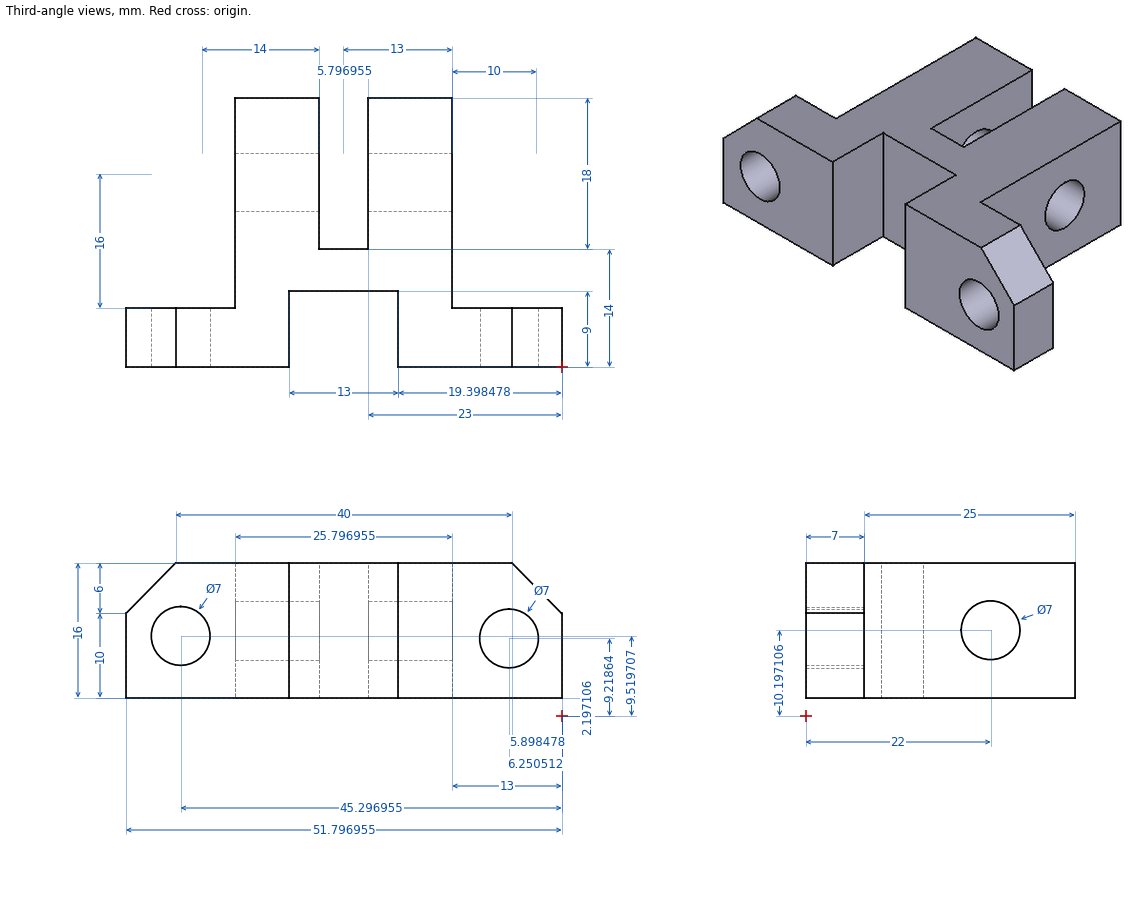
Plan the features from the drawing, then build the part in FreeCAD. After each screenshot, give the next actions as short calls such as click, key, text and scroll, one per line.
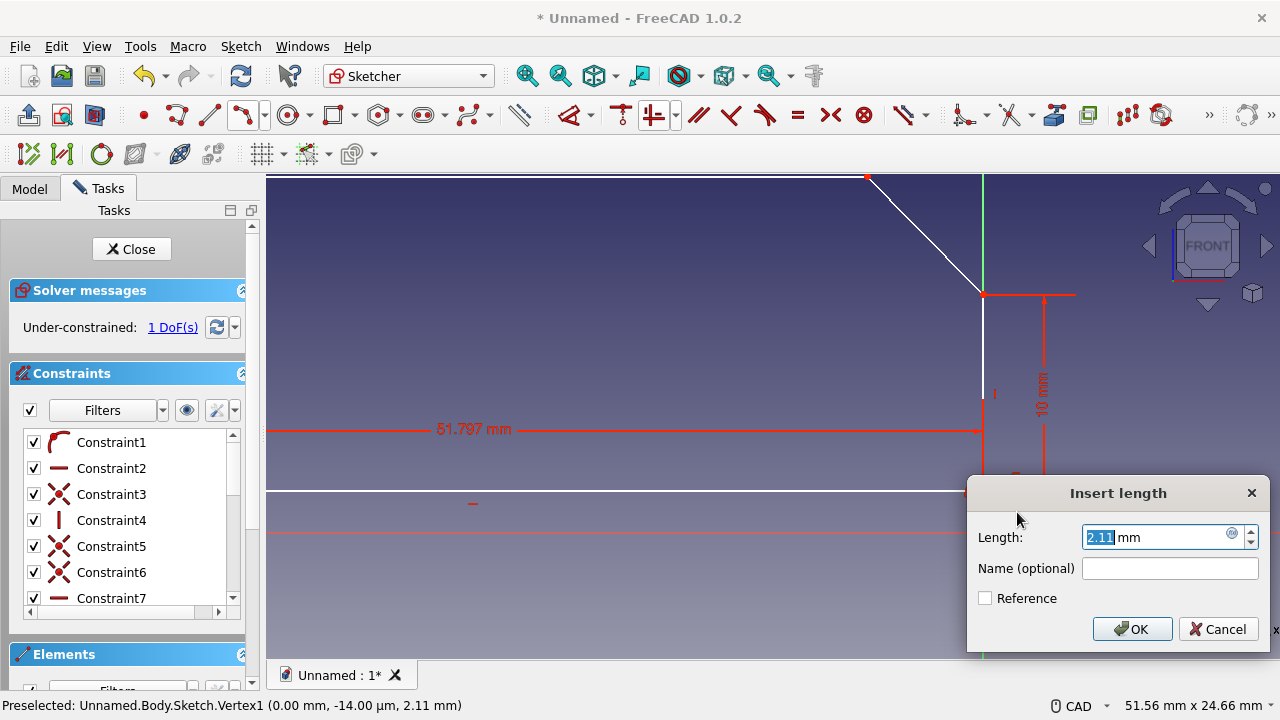
text(2.197106)
key(Return)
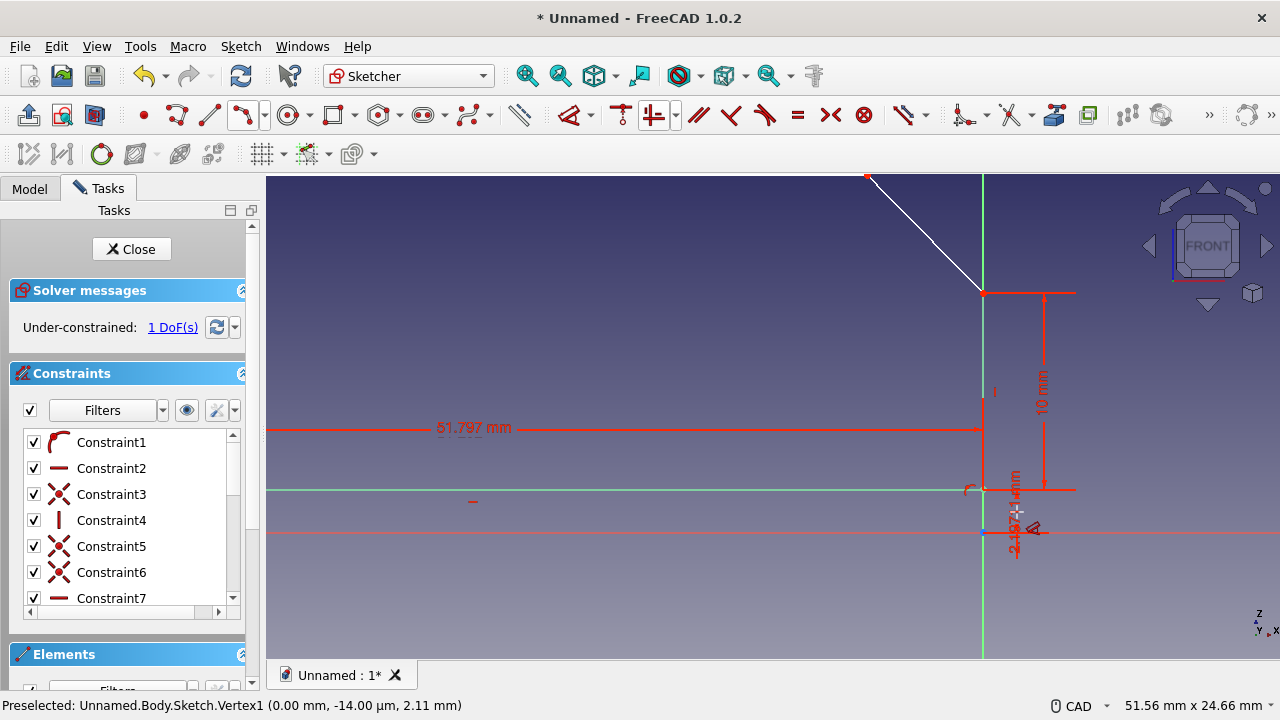
scroll(985, 493, down, 3)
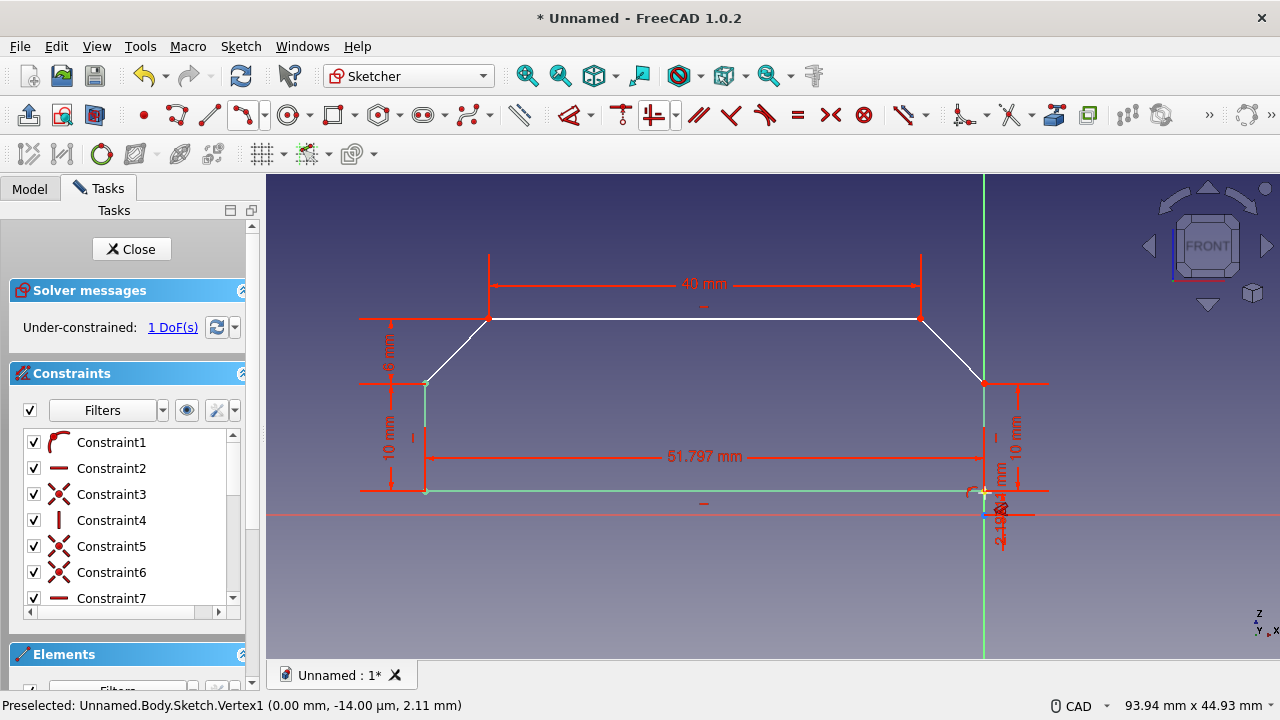
click(921, 319)
click(952, 549)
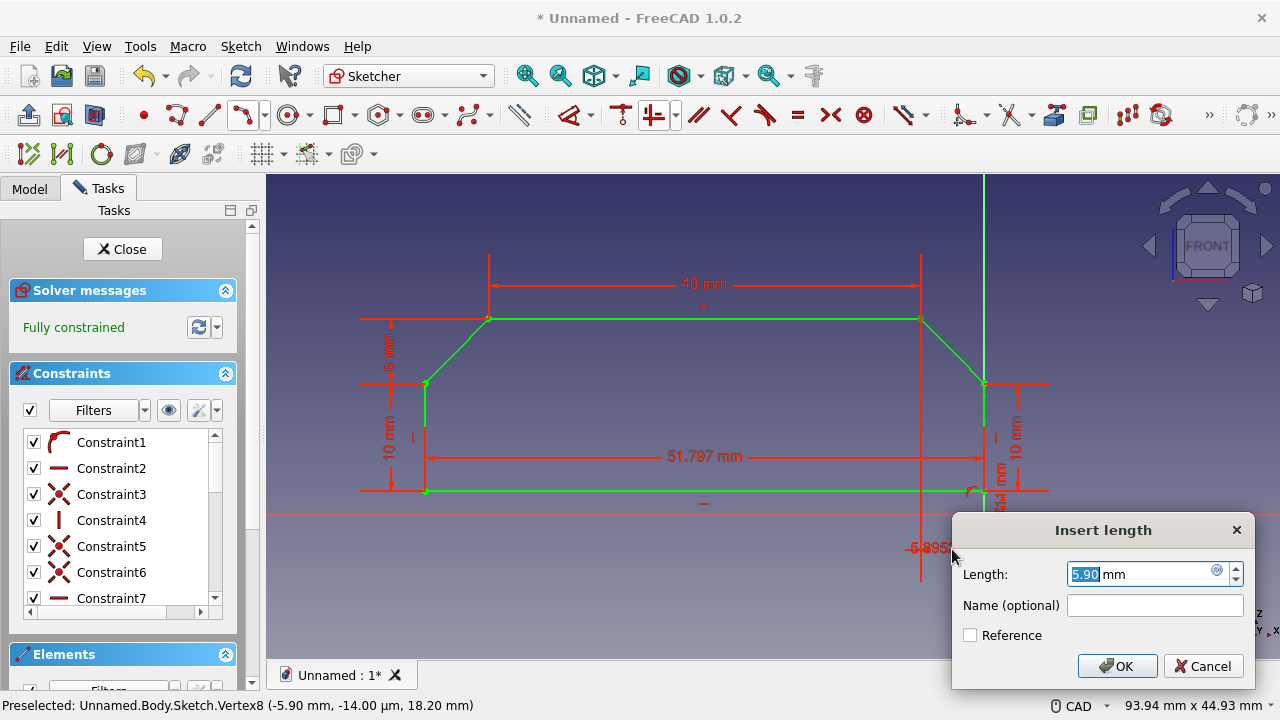
text(5.898478)
key(Return)
key(Escape)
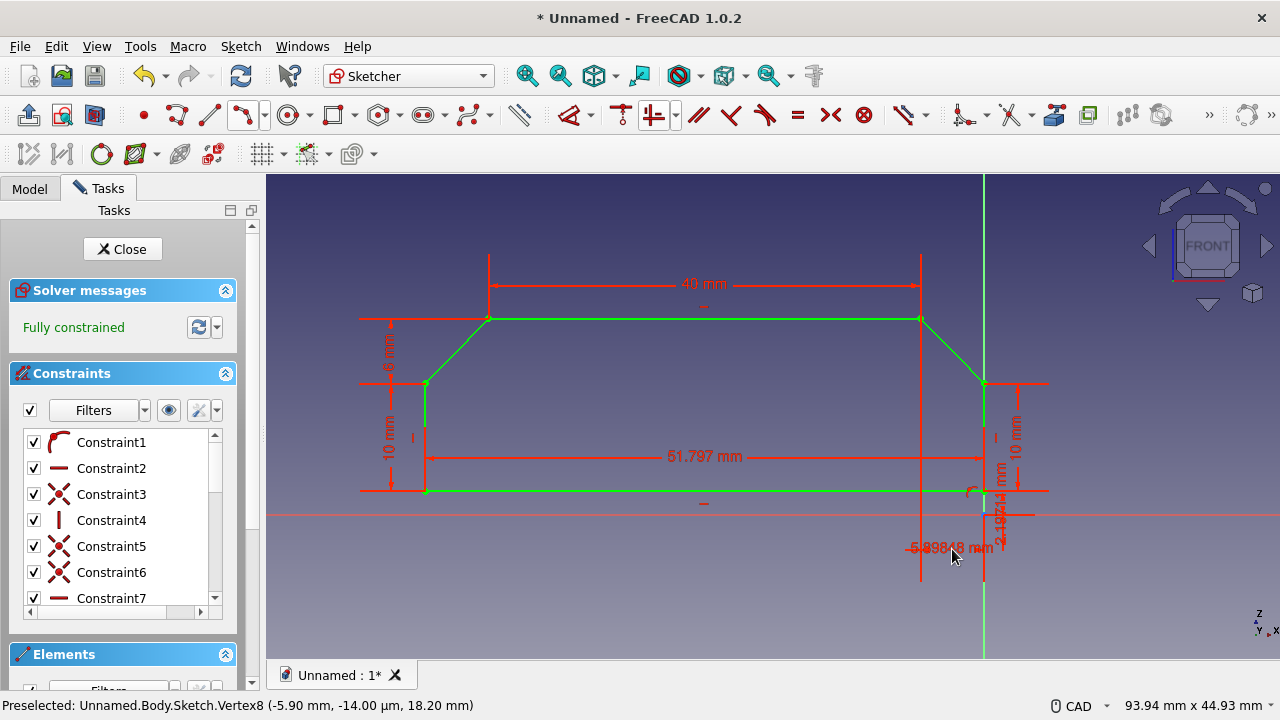
click(123, 249)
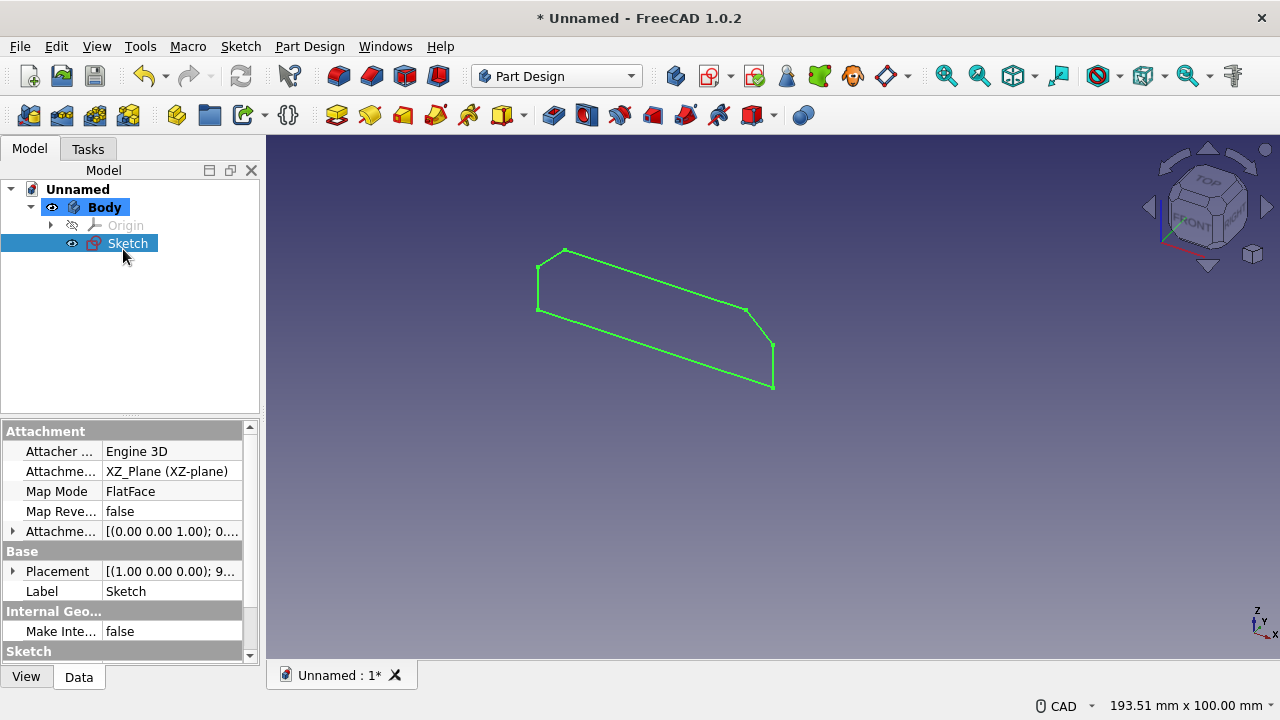
click(337, 116)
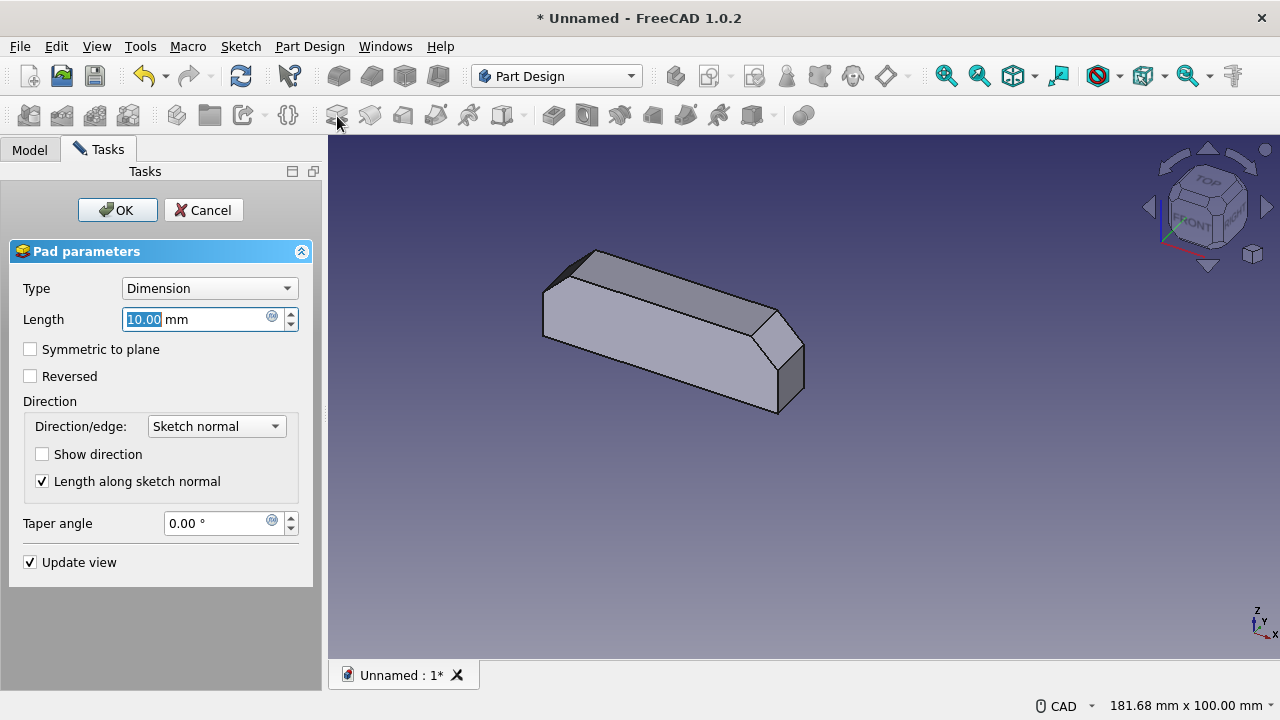
text(7)
key(Tab)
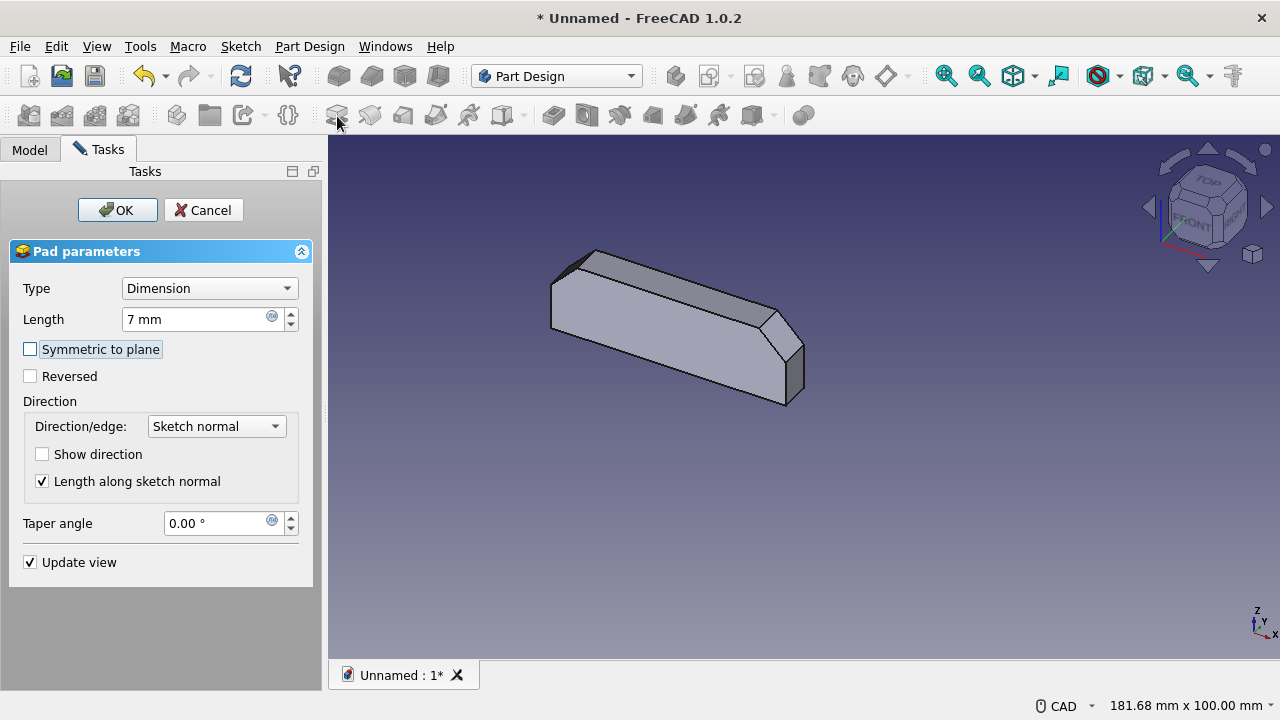
click(31, 376)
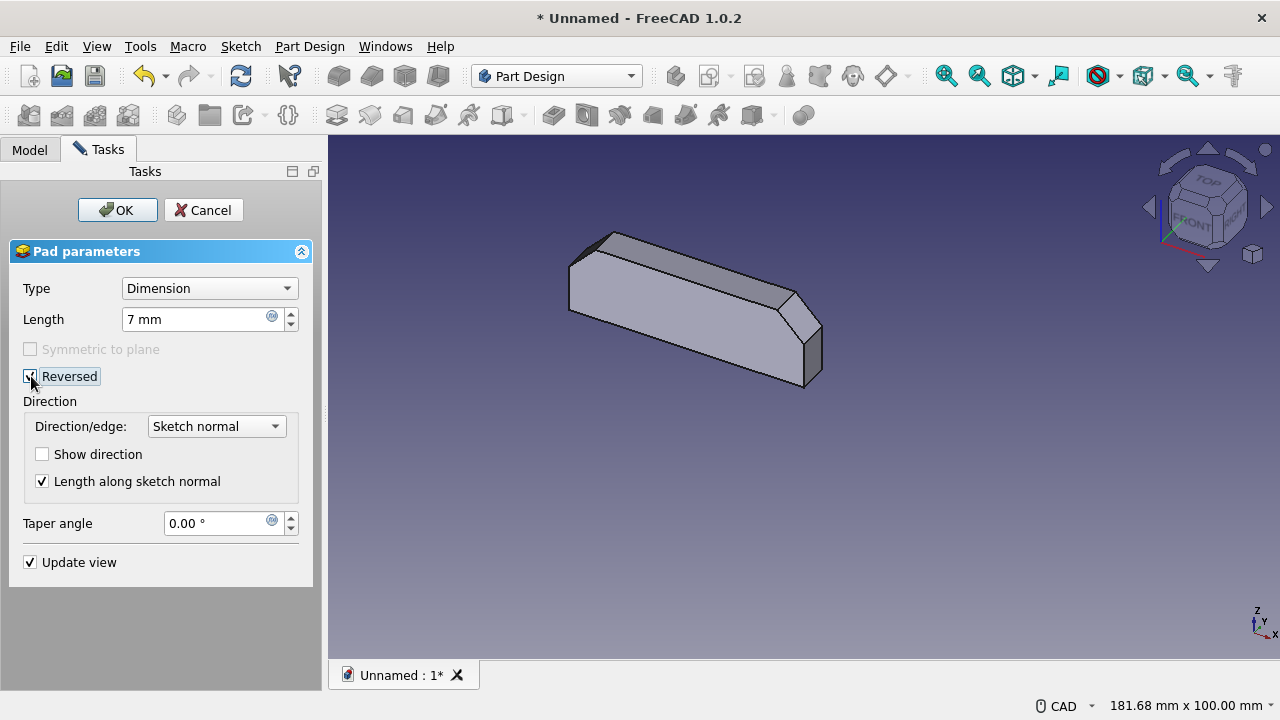
click(118, 210)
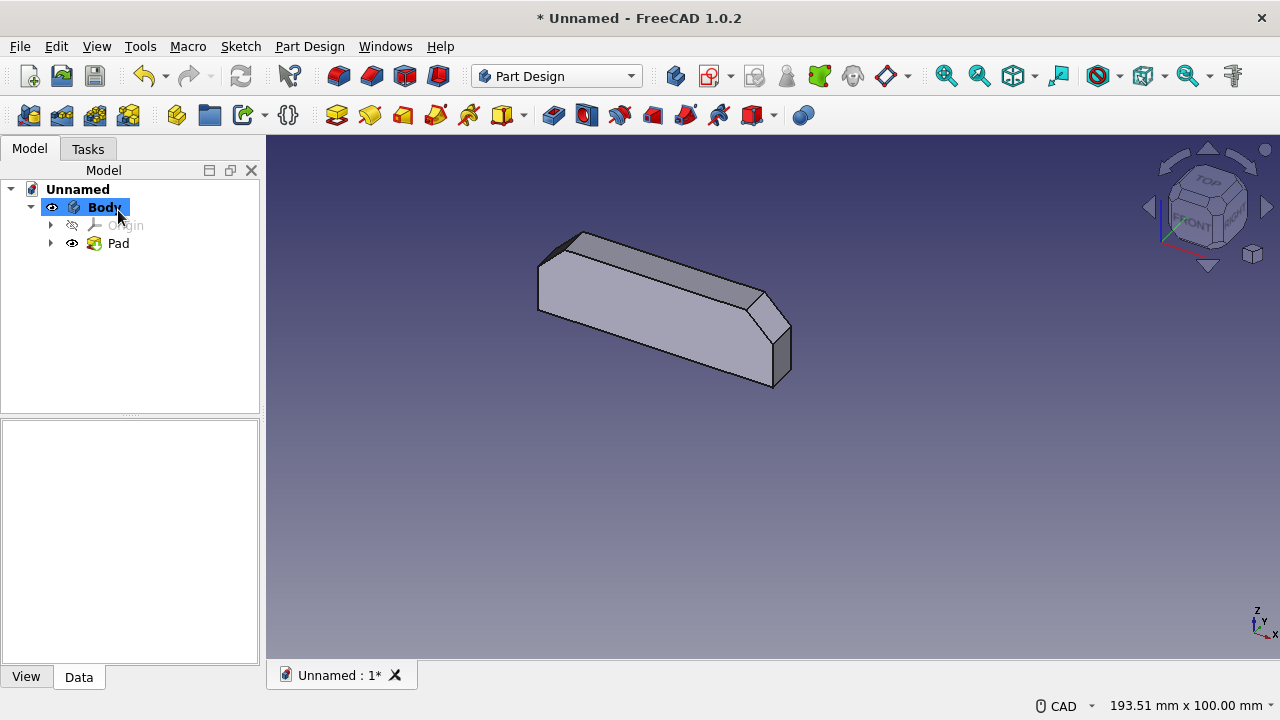
click(947, 76)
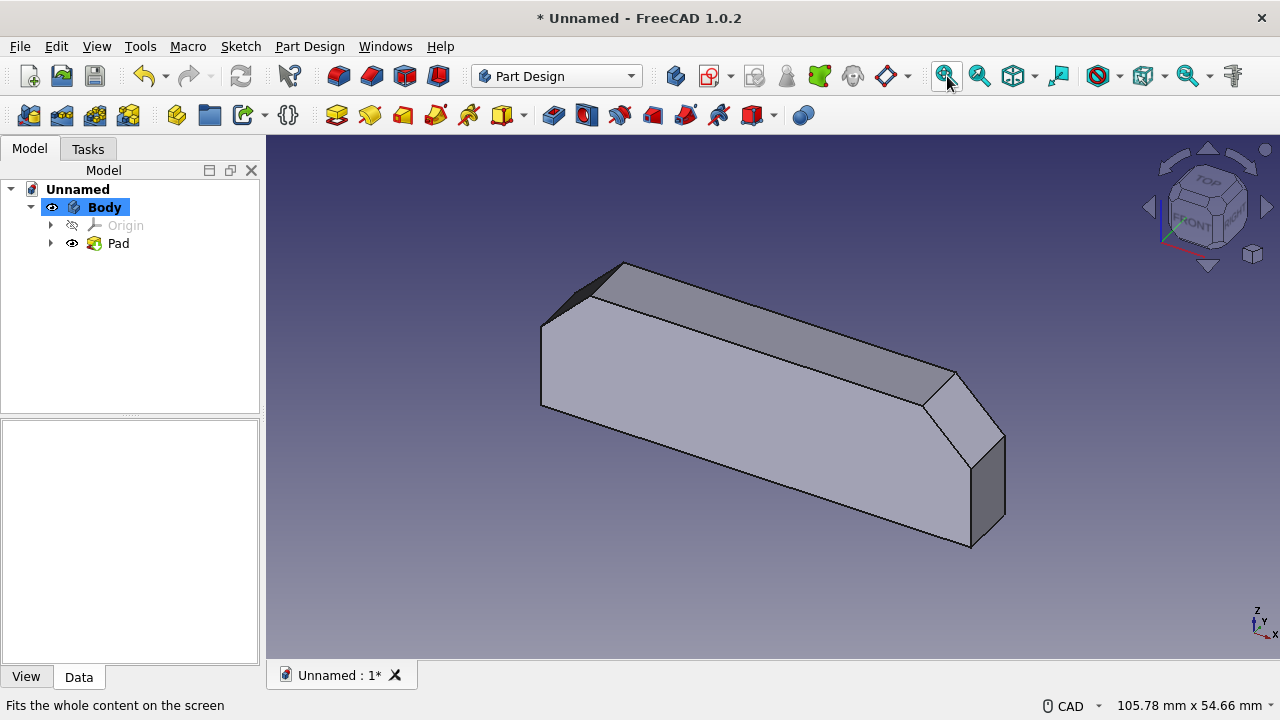
key(4)